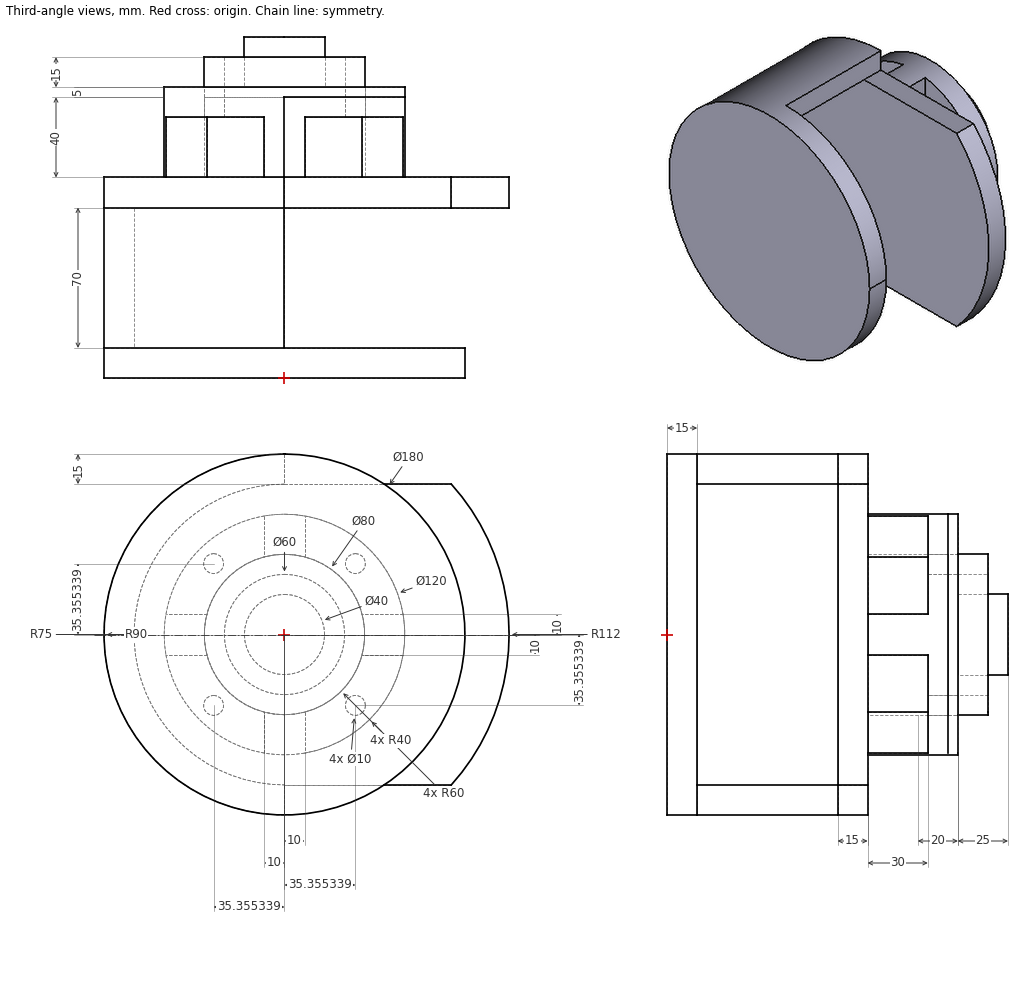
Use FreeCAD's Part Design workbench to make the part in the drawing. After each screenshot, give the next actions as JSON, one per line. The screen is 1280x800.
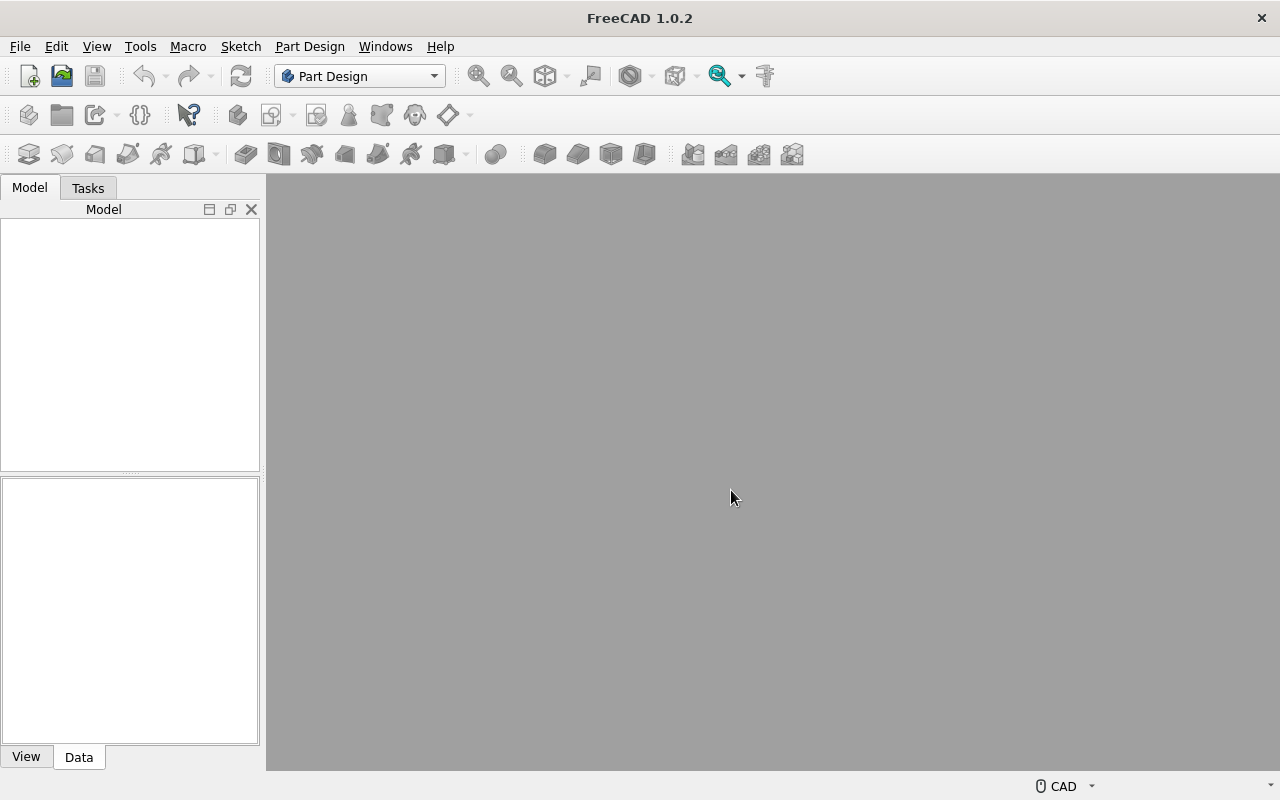
{"action": "left_click", "coordinate": [29, 76]}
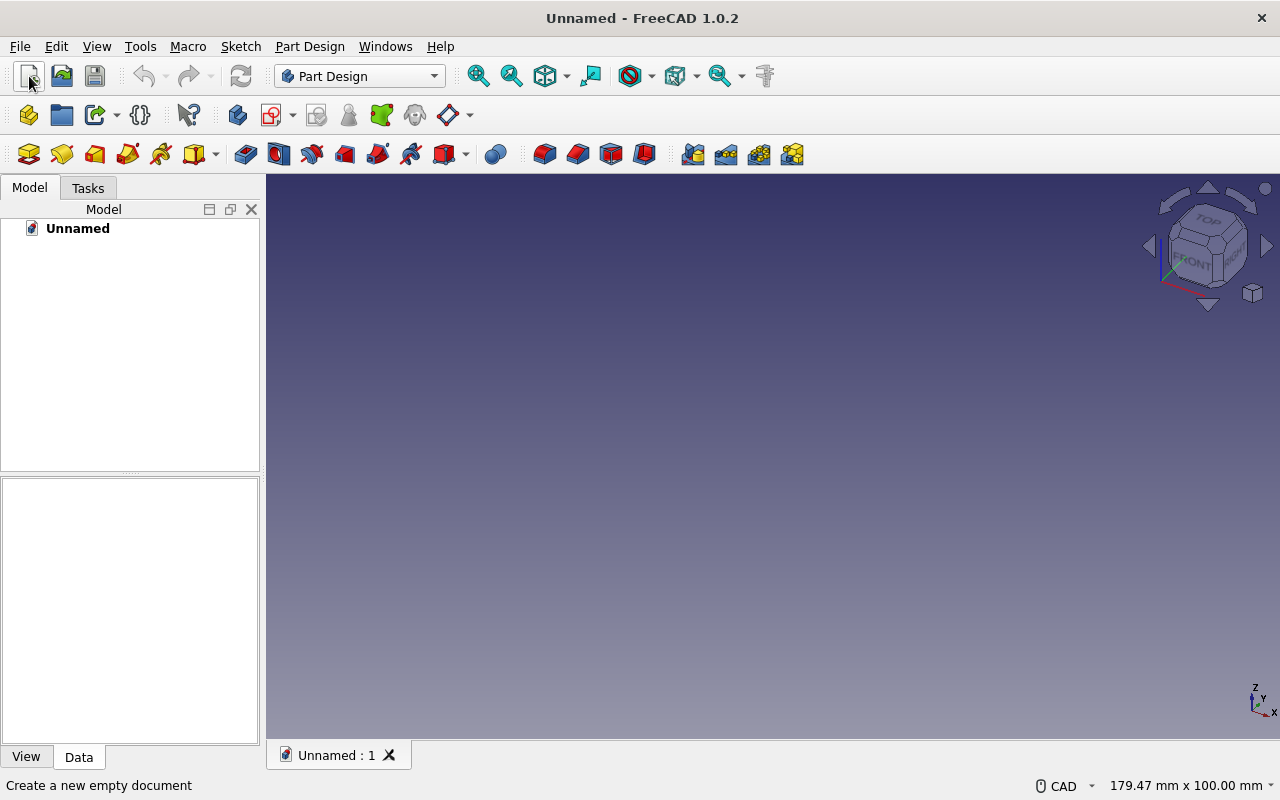
{"action": "left_click", "coordinate": [270, 116]}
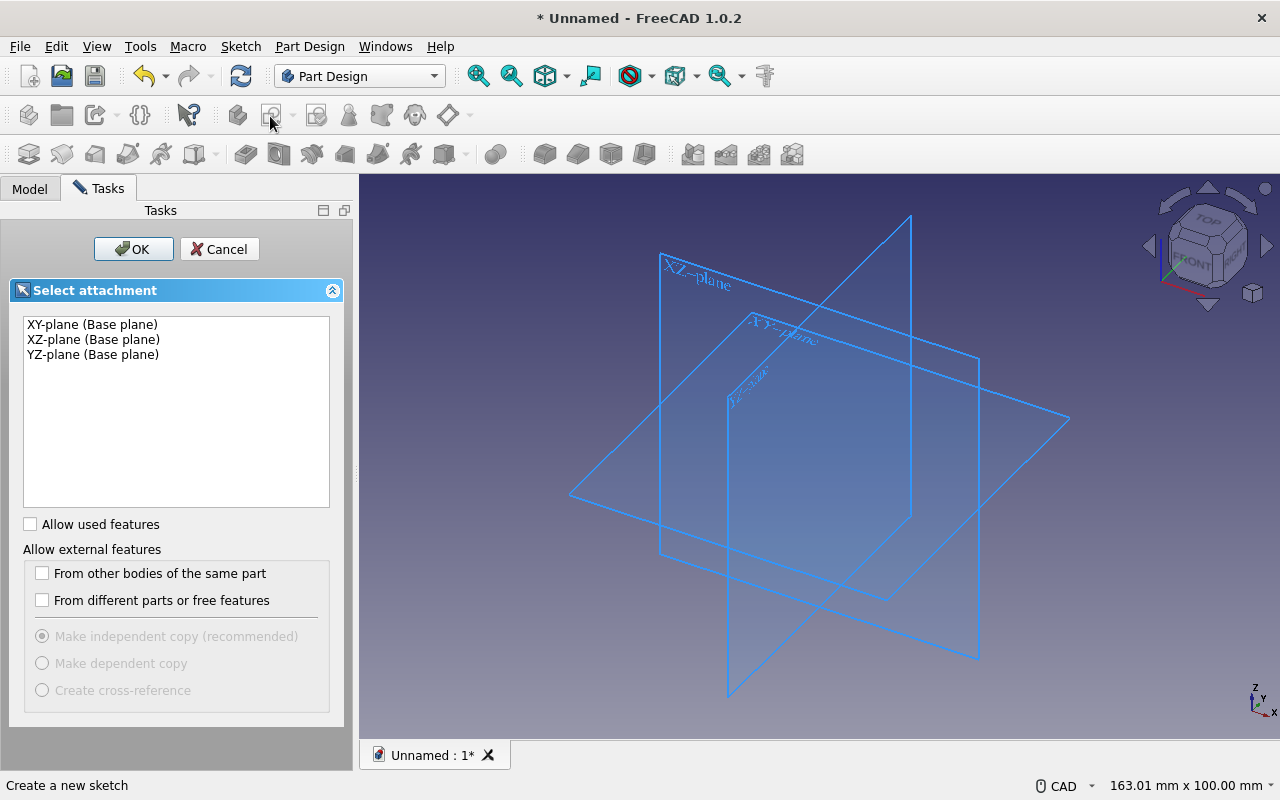
{"action": "left_click", "coordinate": [84, 340]}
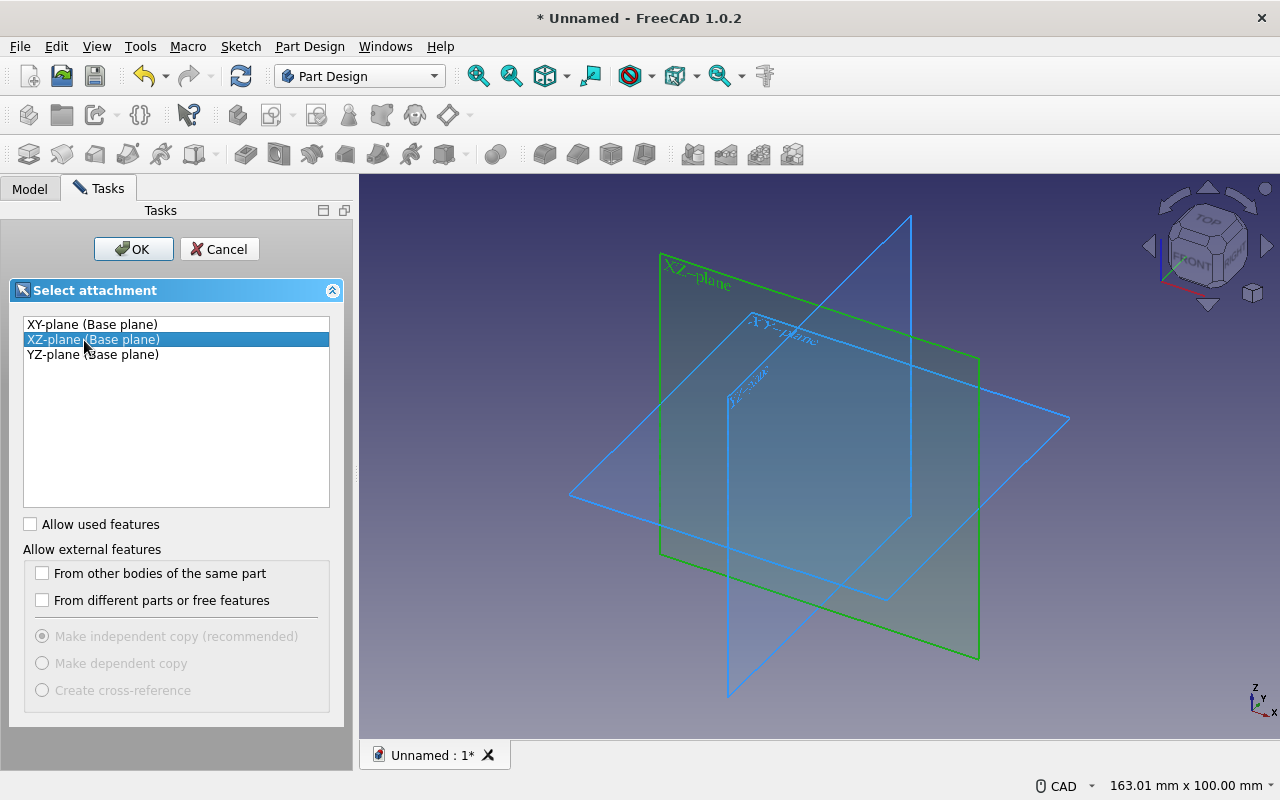
{"action": "left_click", "coordinate": [134, 249]}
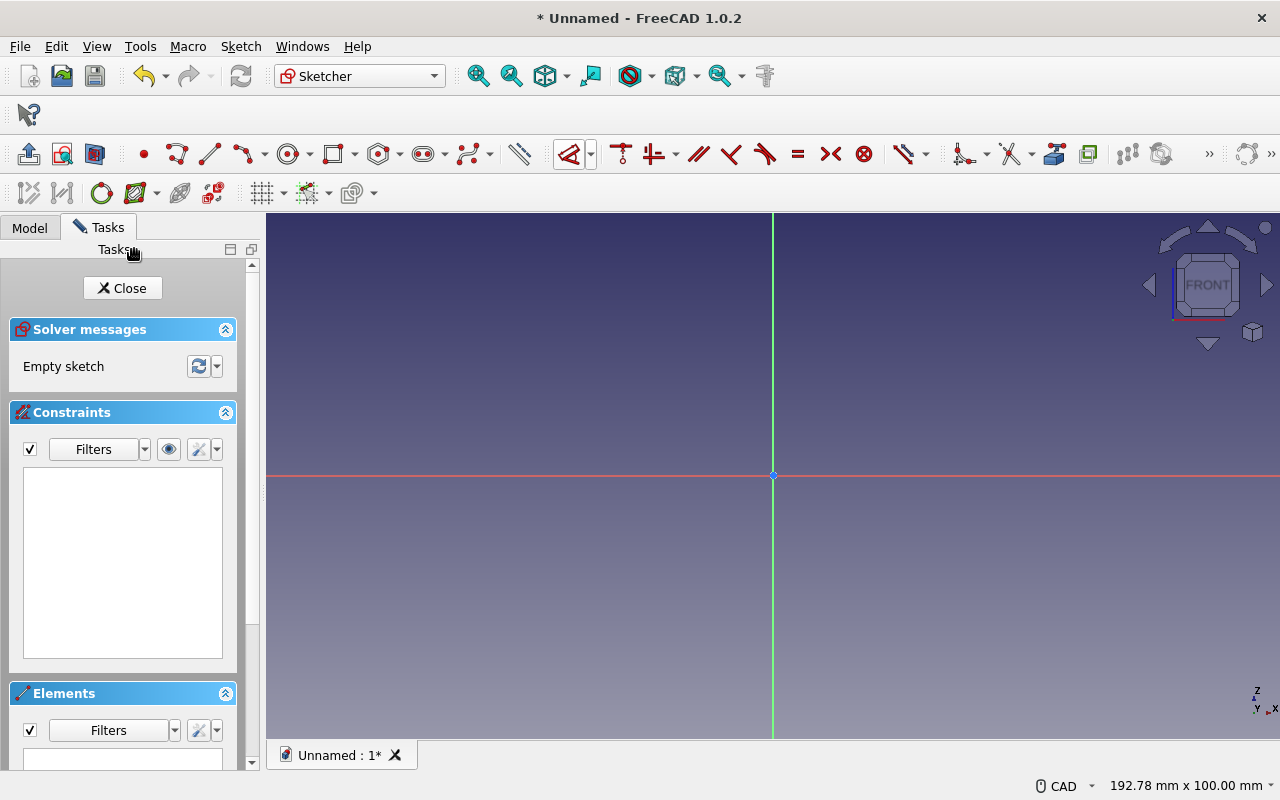
{"action": "scroll", "coordinate": [665, 476], "scroll_direction": "down", "scroll_amount": 5}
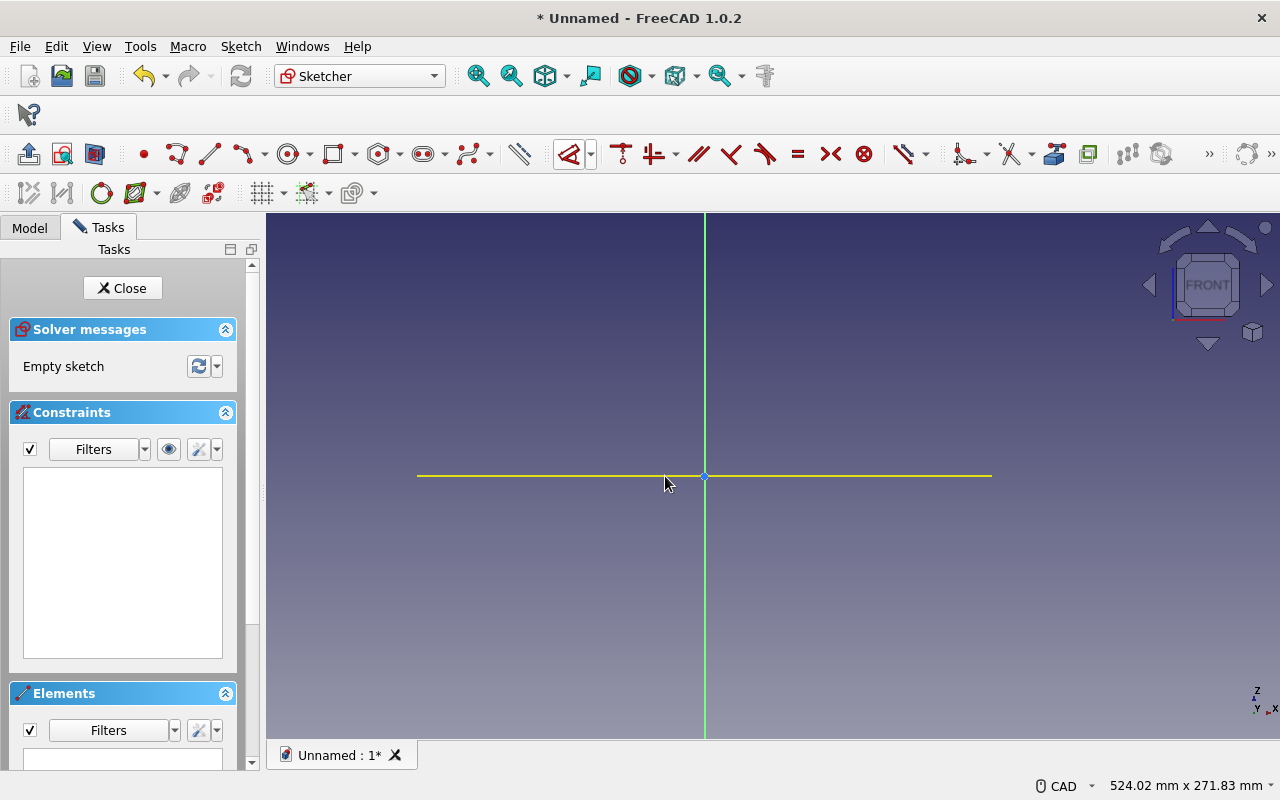
{"action": "left_click", "coordinate": [288, 154]}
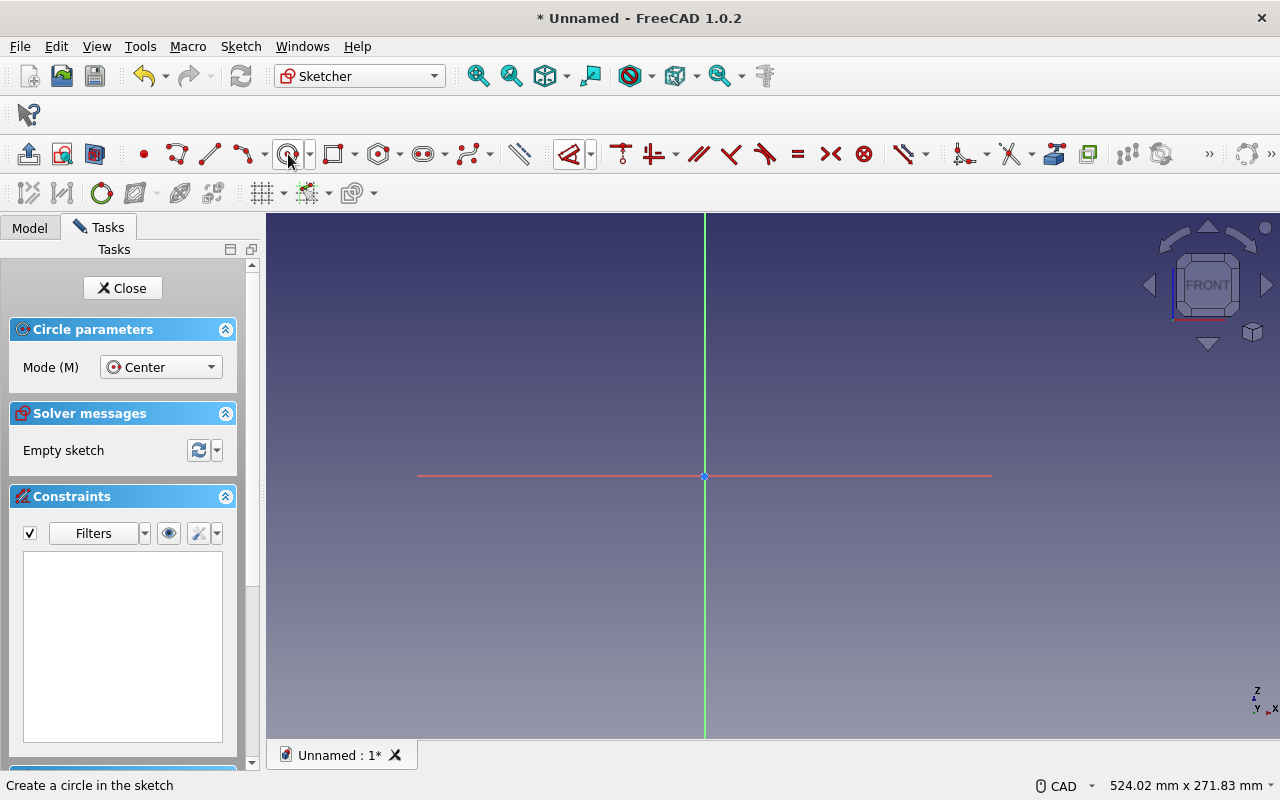
{"action": "left_click", "coordinate": [705, 476]}
{"action": "left_click", "coordinate": [828, 353]}
{"action": "key", "text": "Escape"}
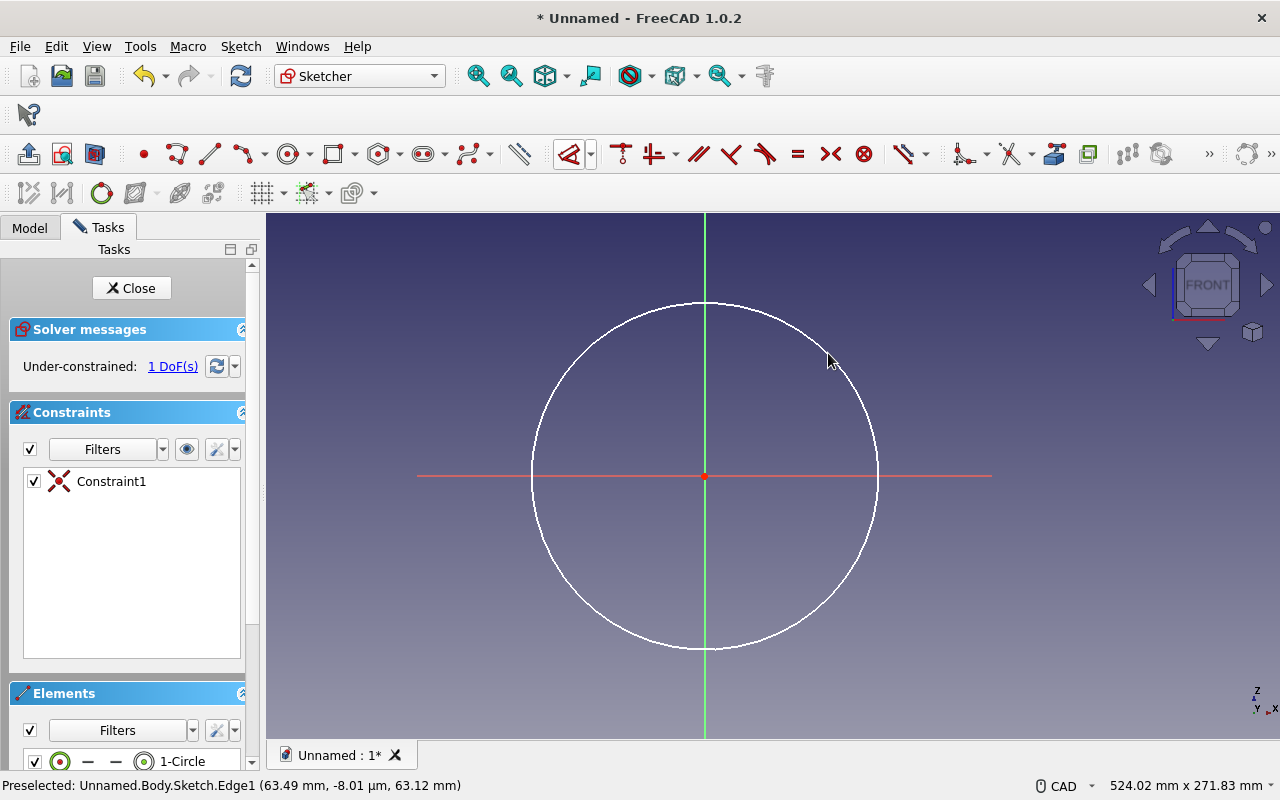
{"action": "left_click", "coordinate": [827, 353]}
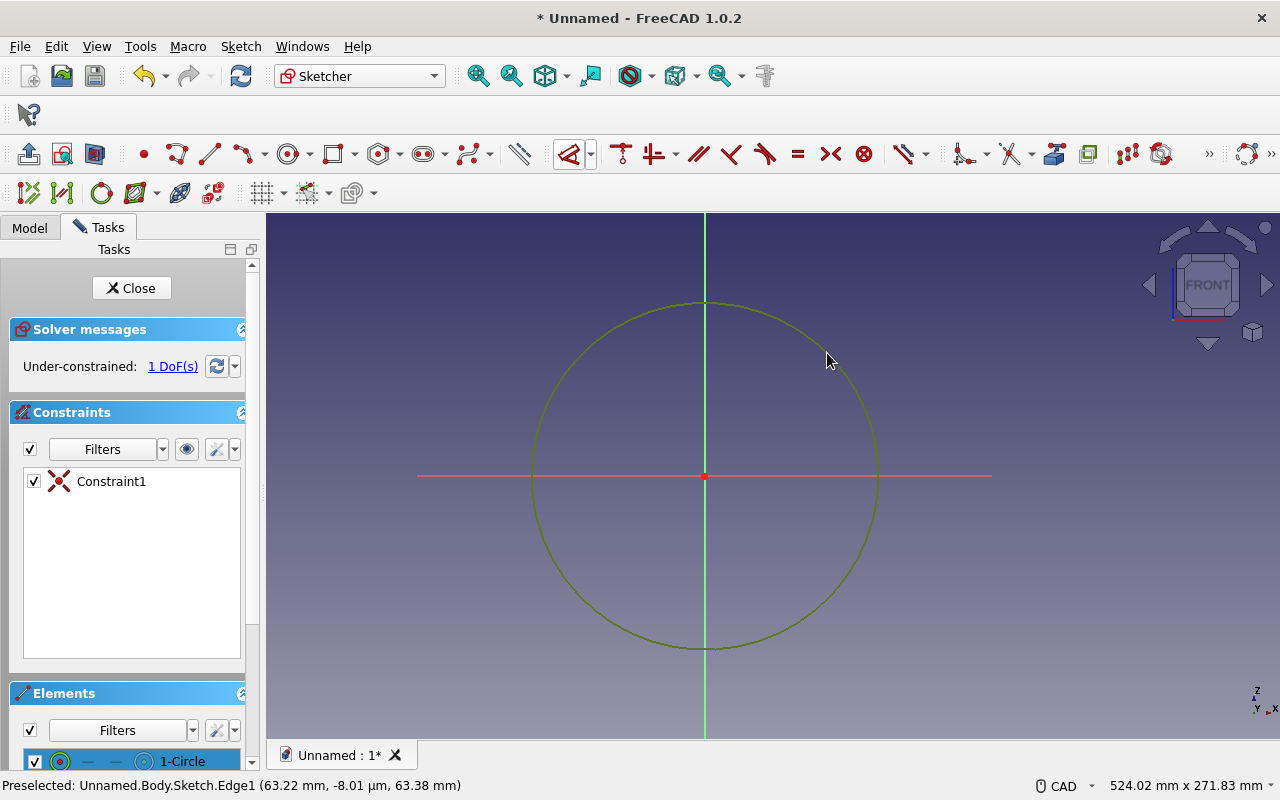
{"action": "left_click", "coordinate": [590, 154]}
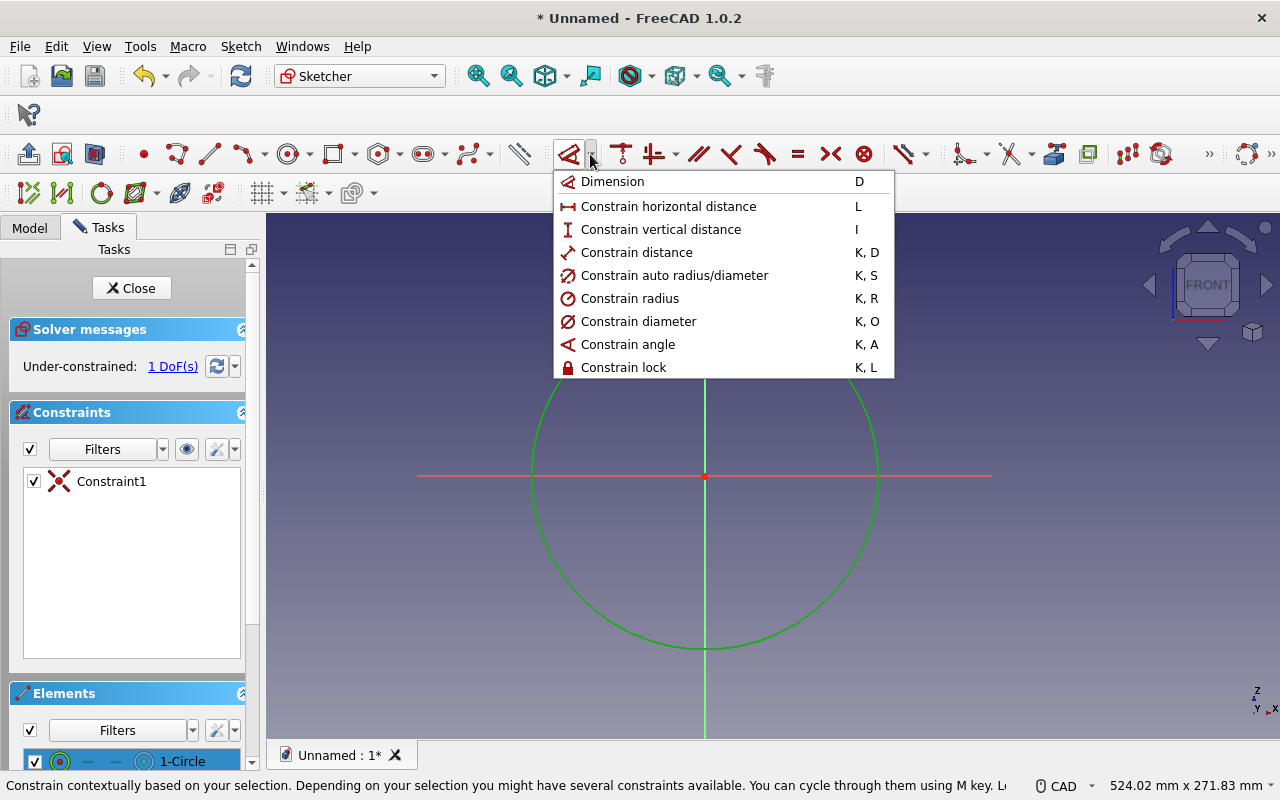
{"action": "left_click", "coordinate": [724, 322]}